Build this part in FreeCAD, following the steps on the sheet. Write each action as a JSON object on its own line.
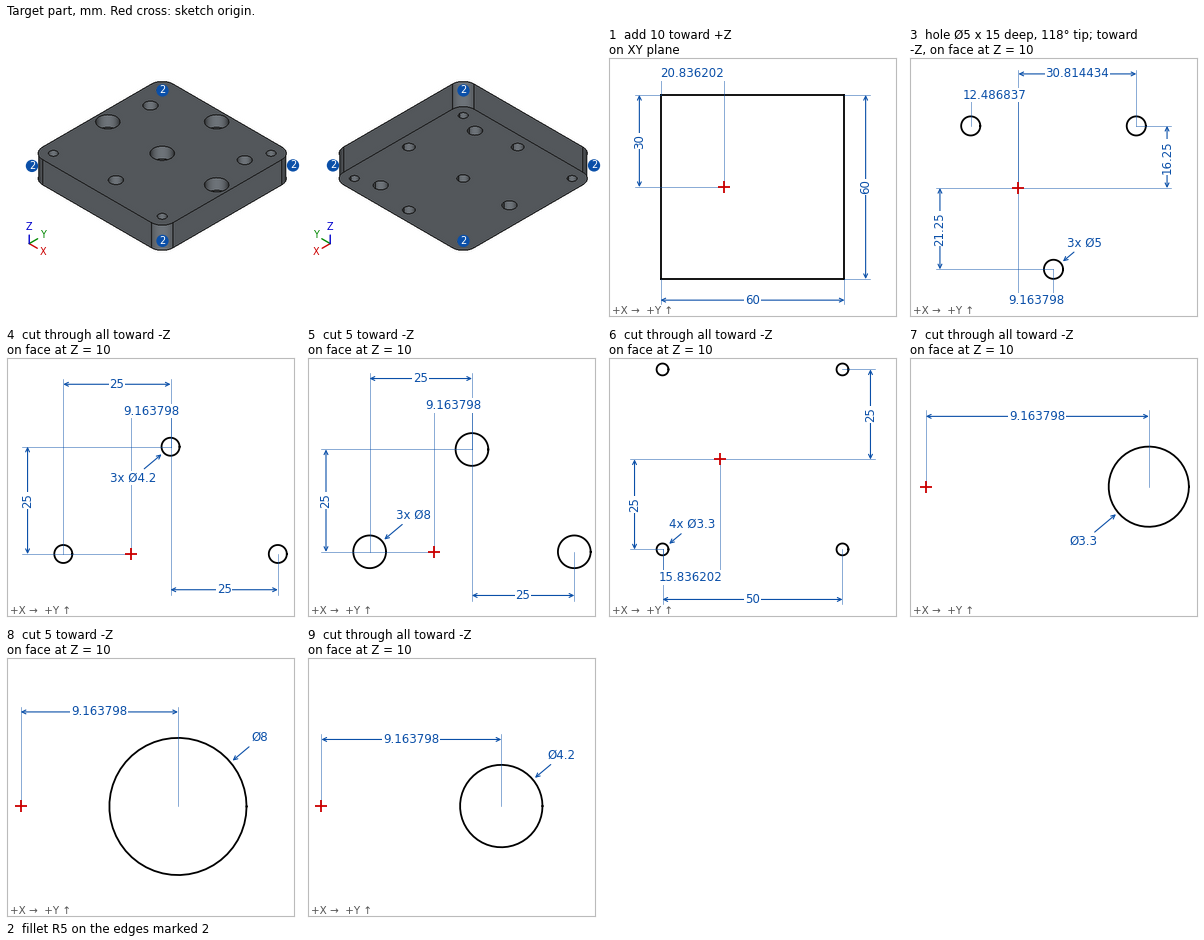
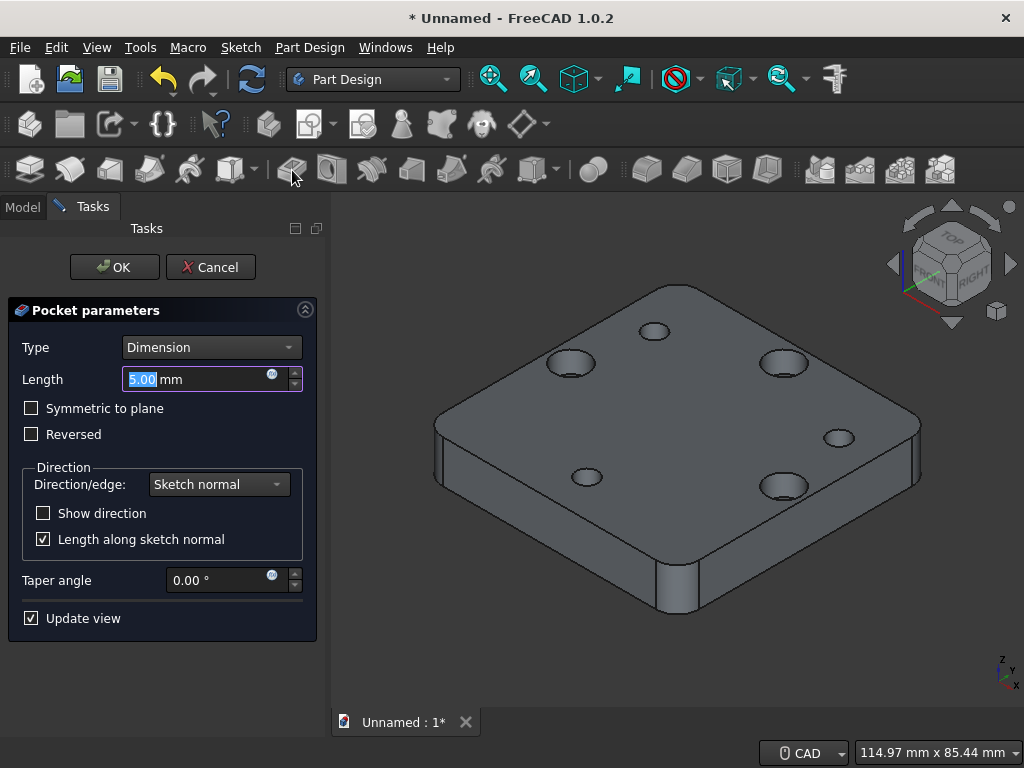
{"action": "type", "text": "5"}
{"action": "key", "text": "Tab"}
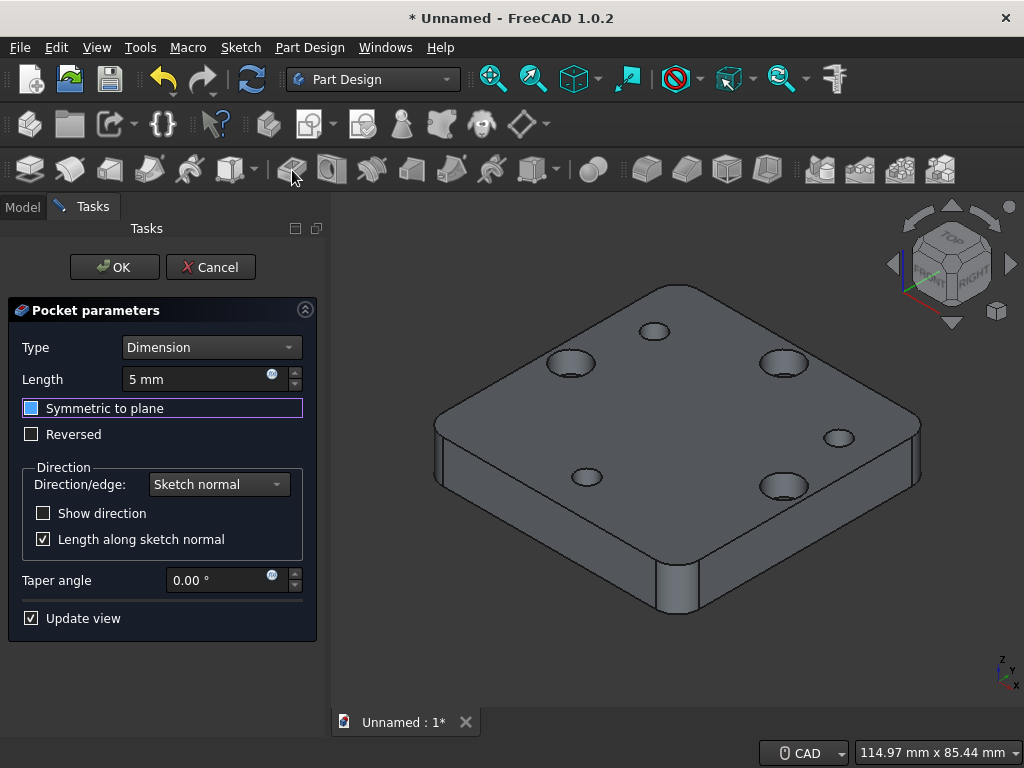
{"action": "left_click", "coordinate": [115, 267]}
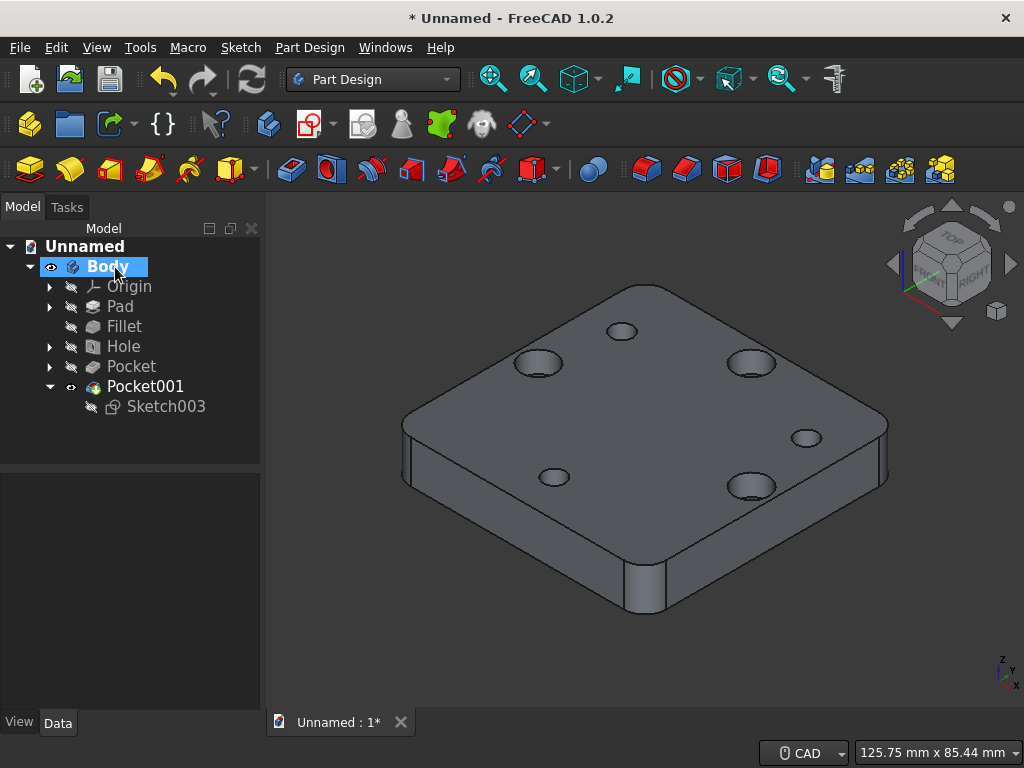
{"action": "left_click", "coordinate": [645, 424]}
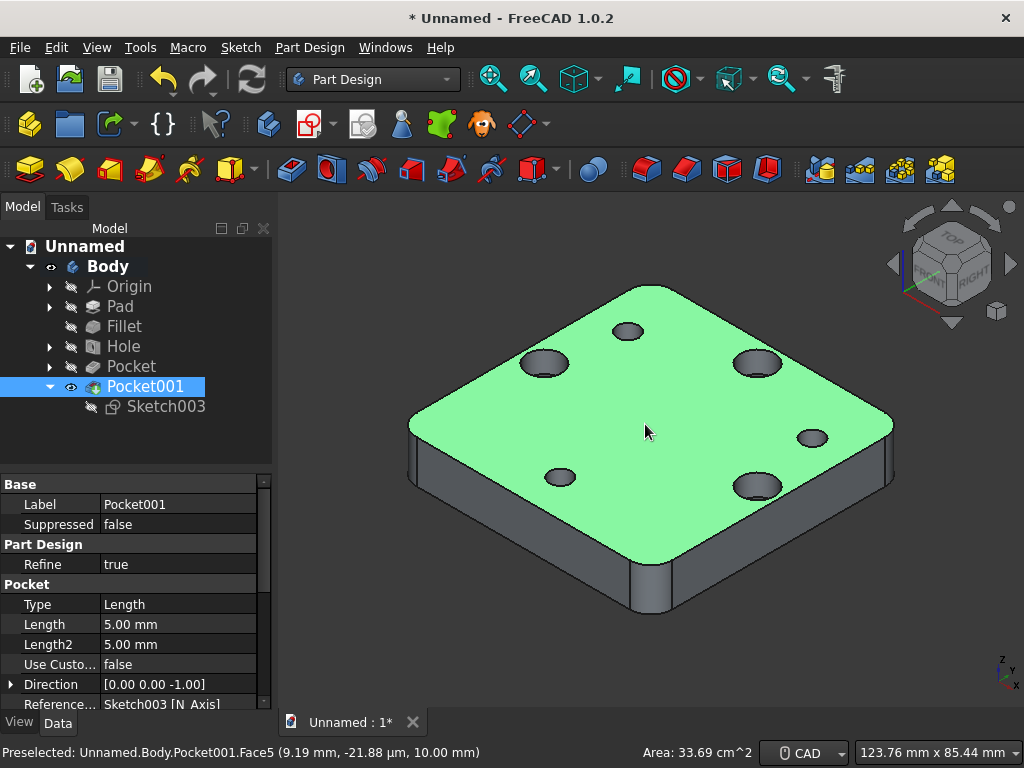
{"action": "left_click", "coordinate": [310, 124]}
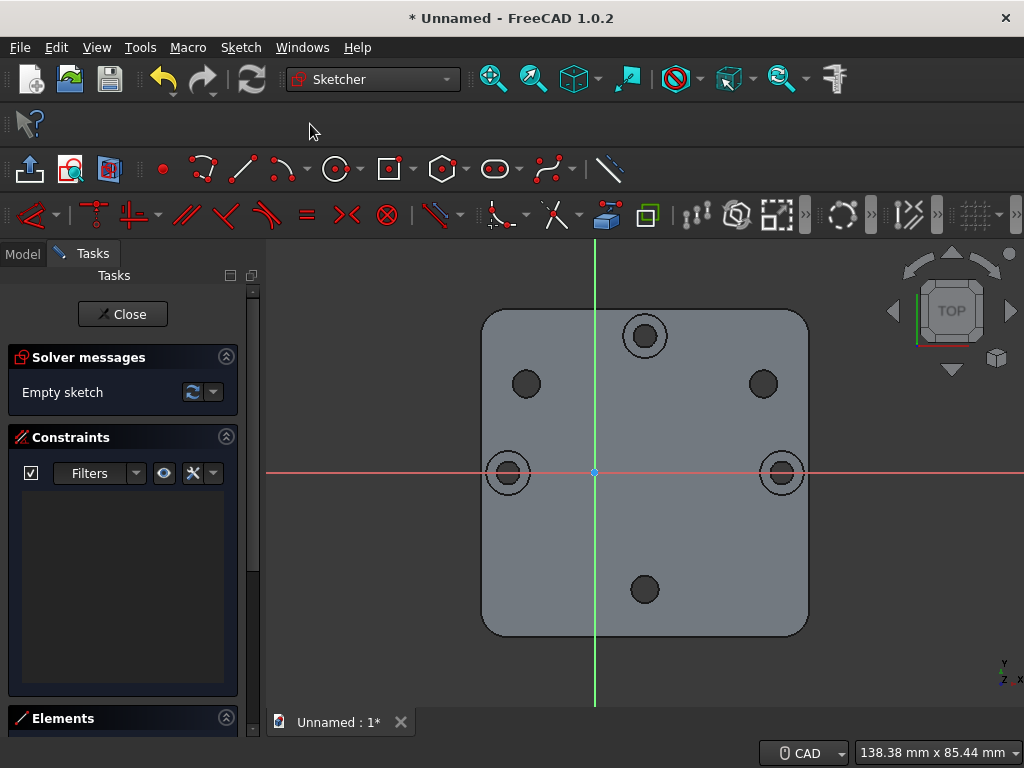
{"action": "left_click", "coordinate": [336, 170]}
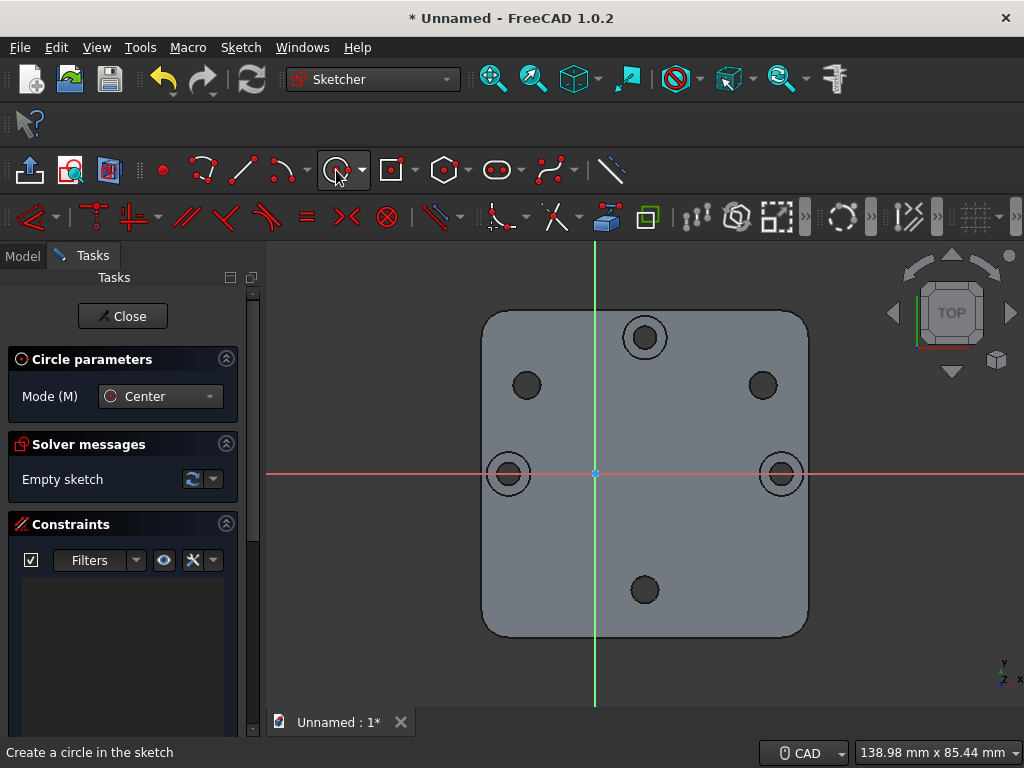
{"action": "scroll", "coordinate": [509, 610], "scroll_direction": "up", "scroll_amount": 5}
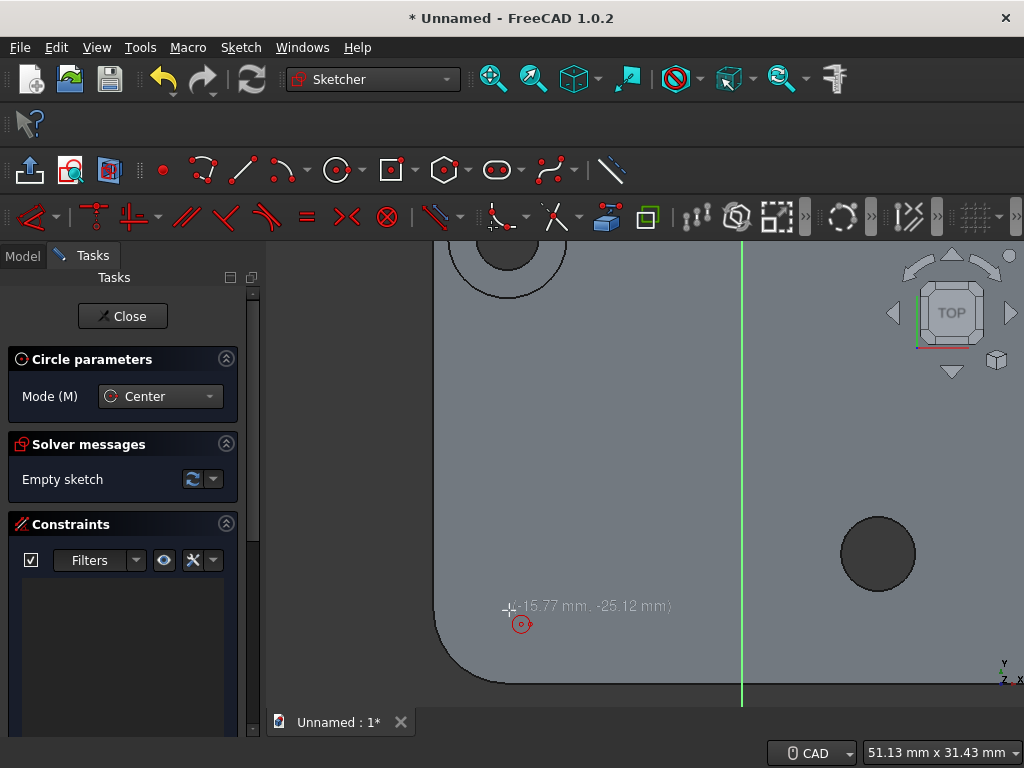
{"action": "left_click", "coordinate": [507, 610]}
{"action": "mouse_move", "coordinate": [525, 592]}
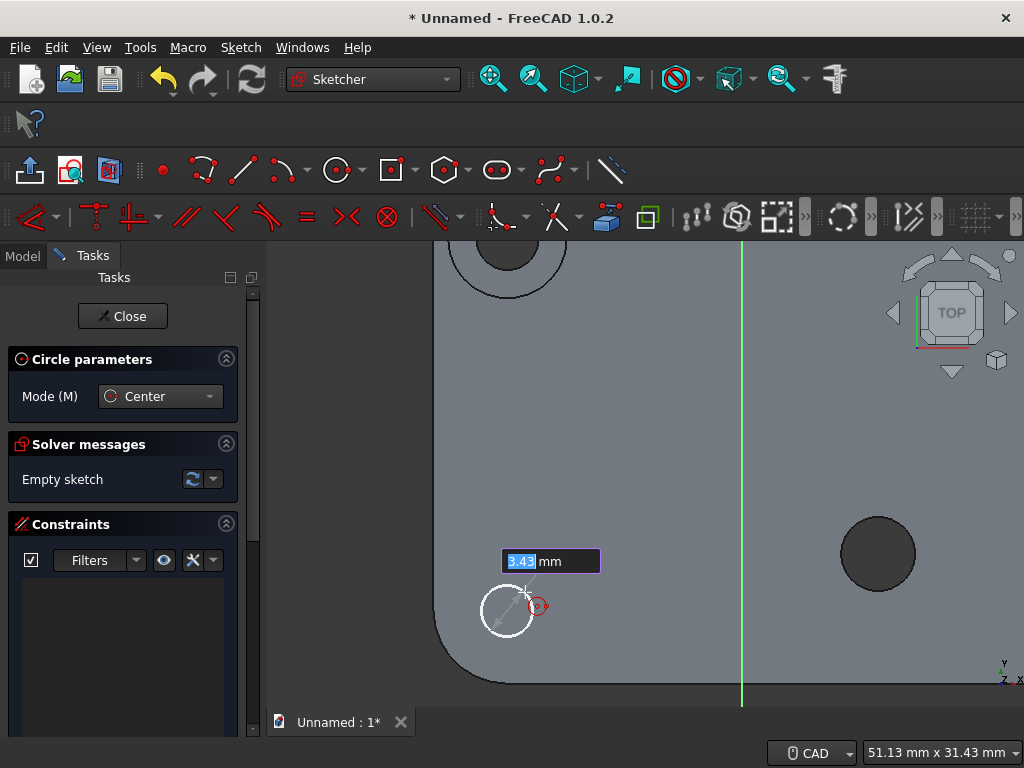
{"action": "type", "text": "3.3"}
{"action": "key", "text": "Return"}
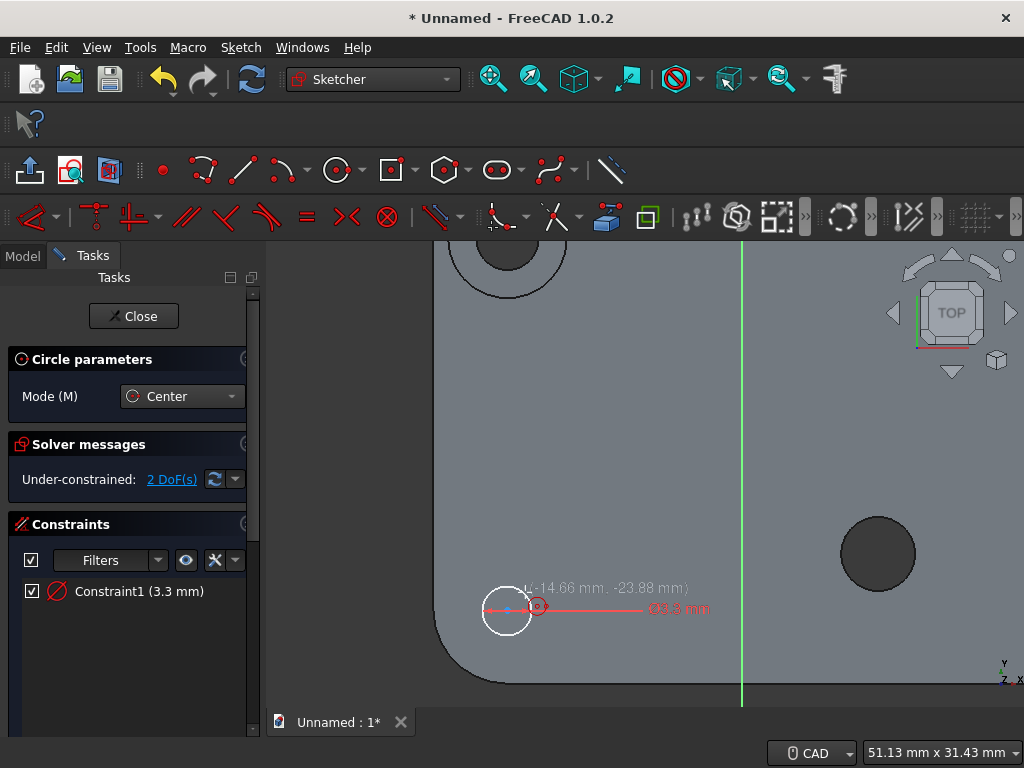
{"action": "scroll", "coordinate": [401, 611], "scroll_direction": "down", "scroll_amount": 5}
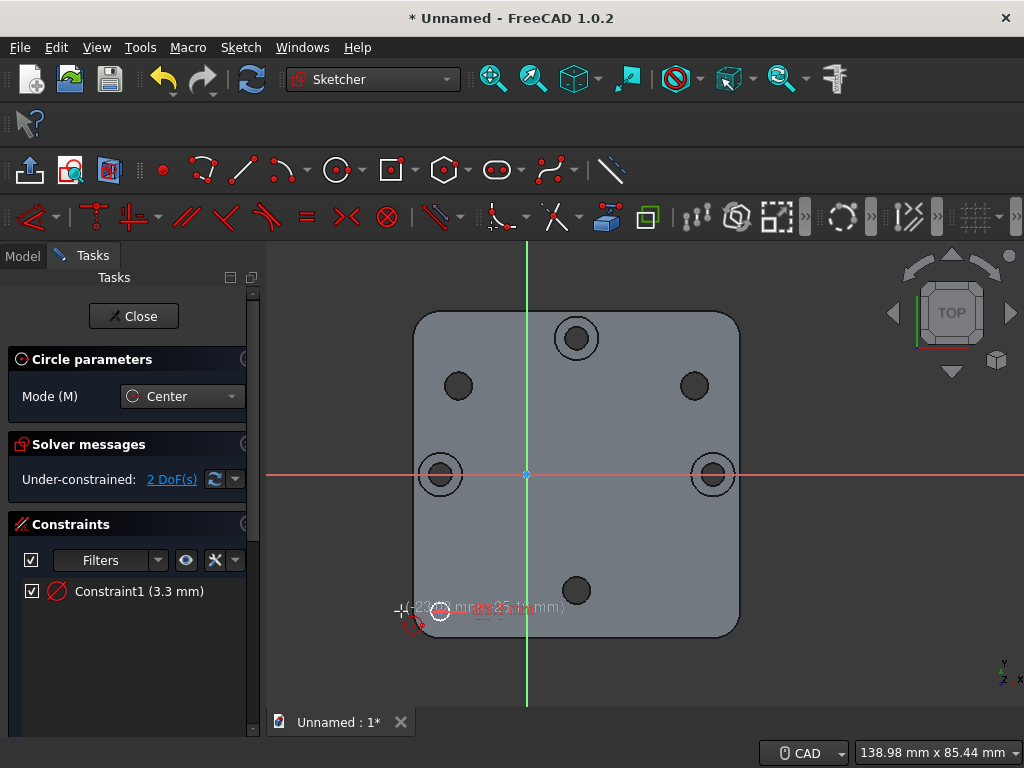
{"action": "scroll", "coordinate": [713, 611], "scroll_direction": "up", "scroll_amount": 5}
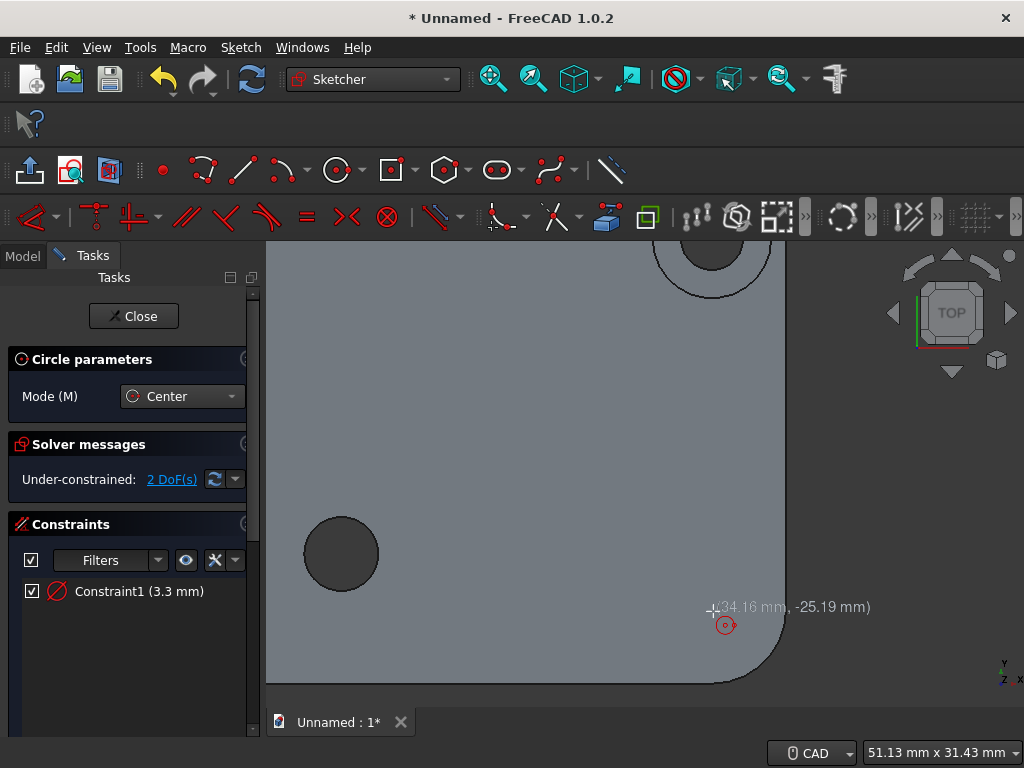
{"action": "left_click", "coordinate": [712, 610]}
{"action": "mouse_move", "coordinate": [729, 592]}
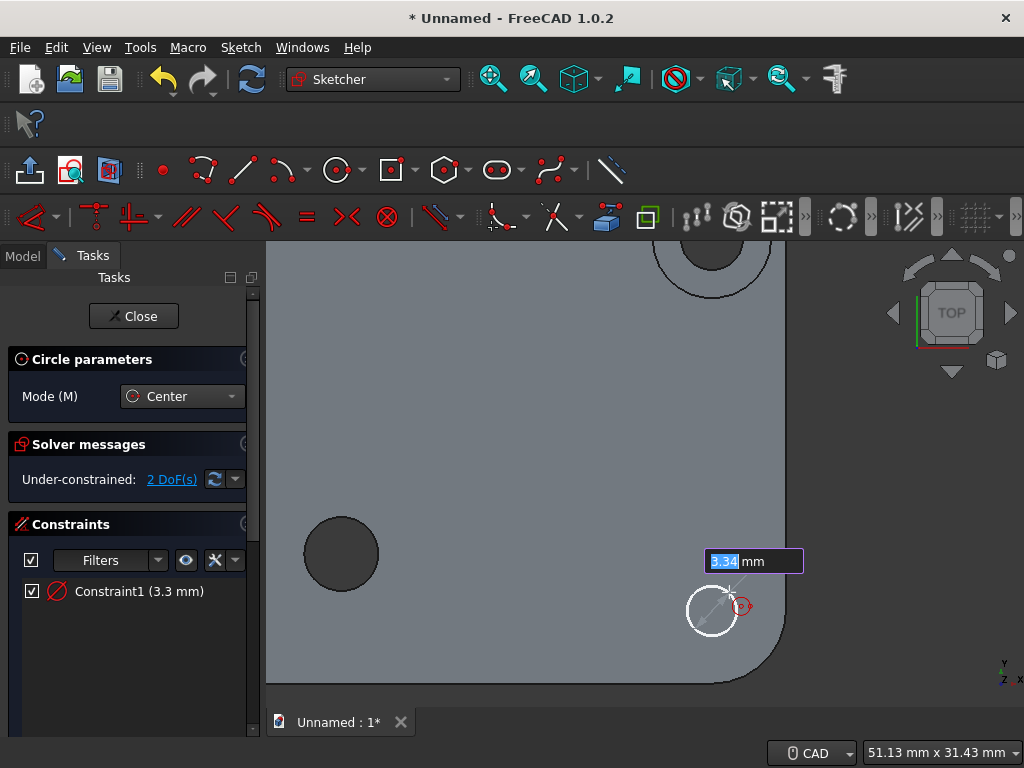
{"action": "type", "text": "3.3"}
{"action": "key", "text": "Return"}